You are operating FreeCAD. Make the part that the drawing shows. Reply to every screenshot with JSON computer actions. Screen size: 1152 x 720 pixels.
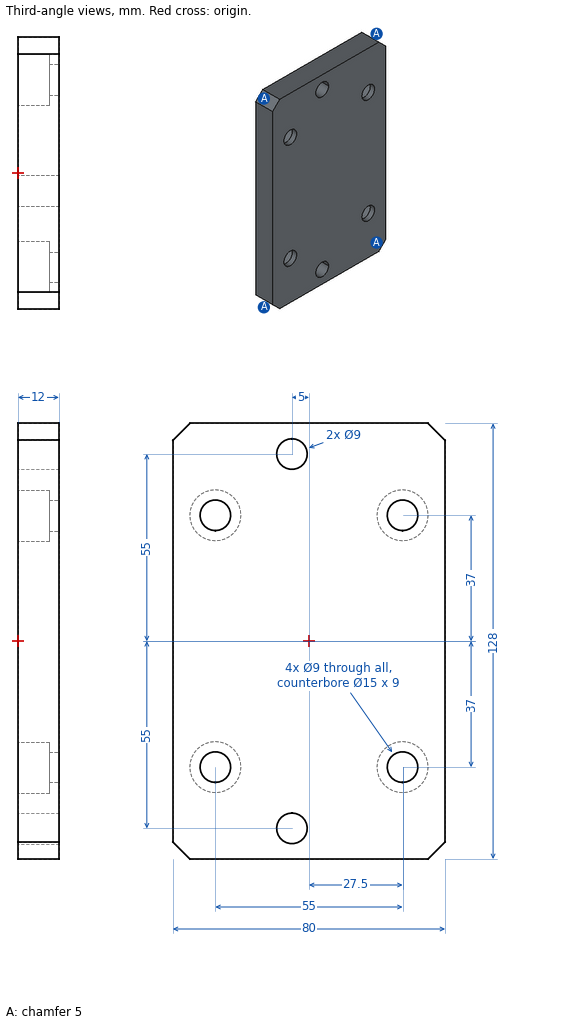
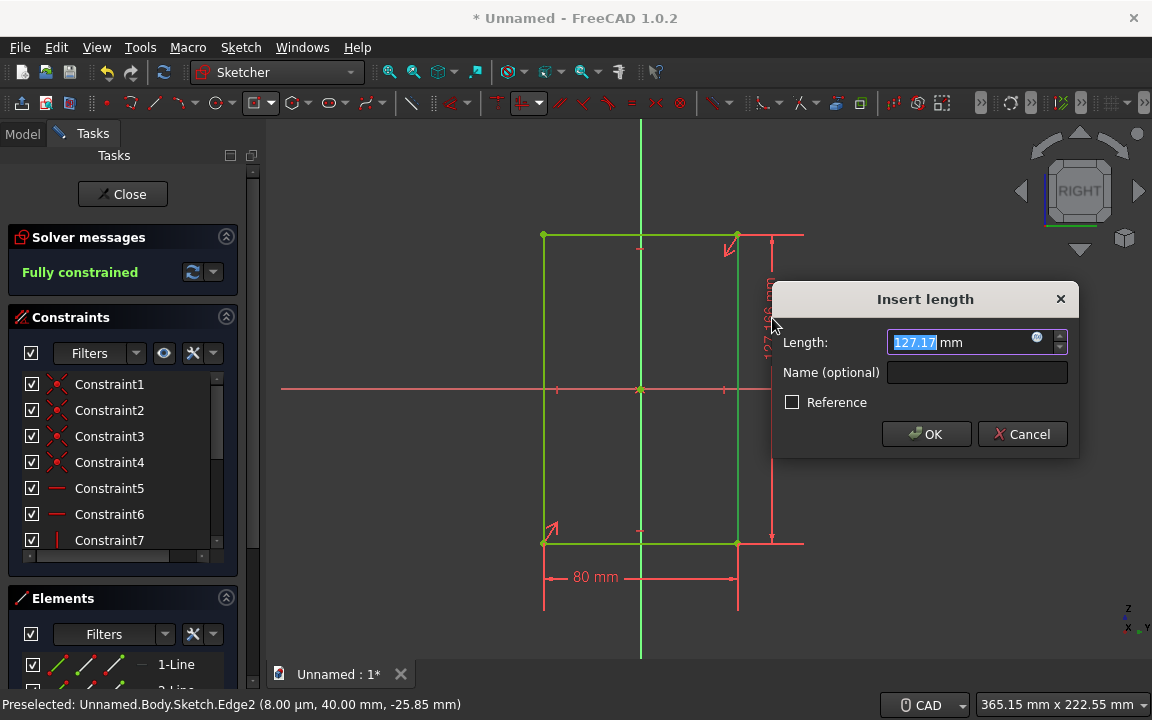
{"action": "type", "text": "128"}
{"action": "key", "text": "Return"}
{"action": "key", "text": "Escape"}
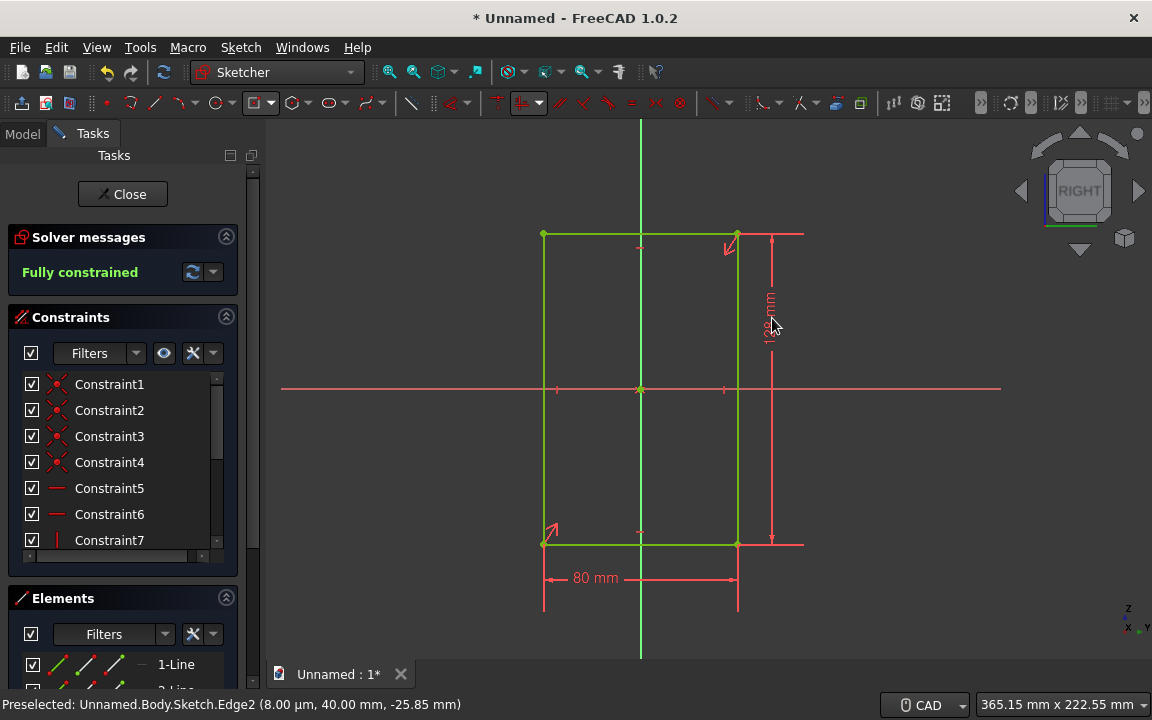
{"action": "left_click", "coordinate": [123, 194]}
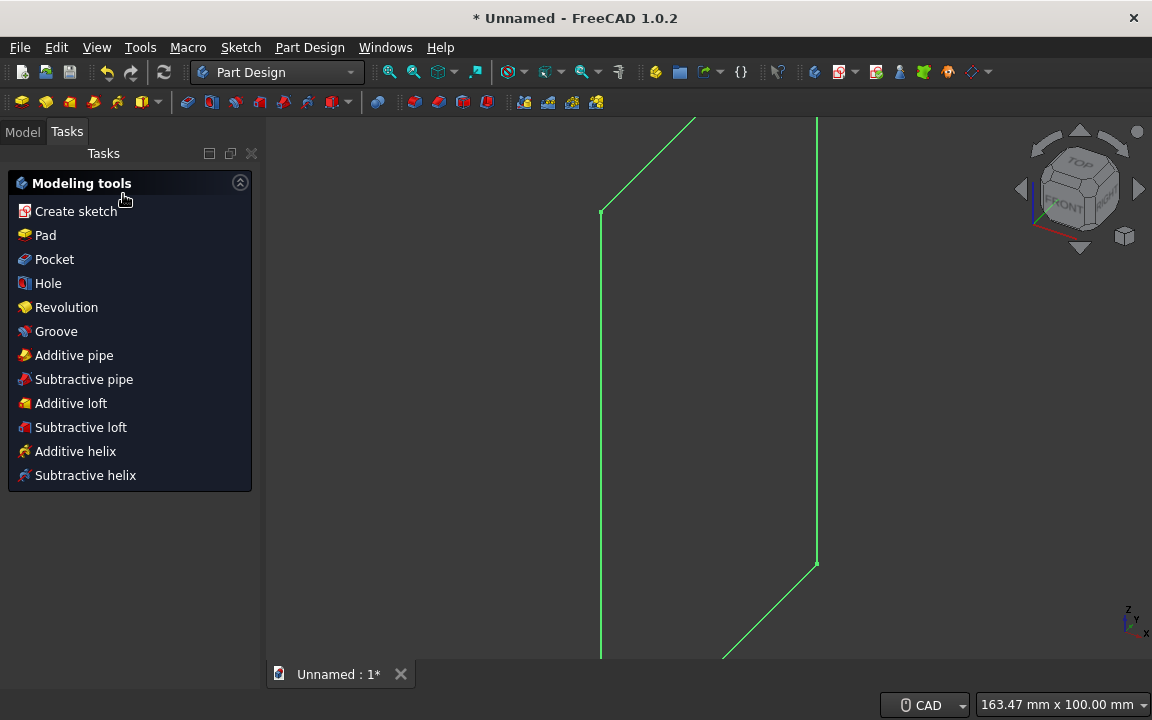
{"action": "left_click", "coordinate": [22, 102]}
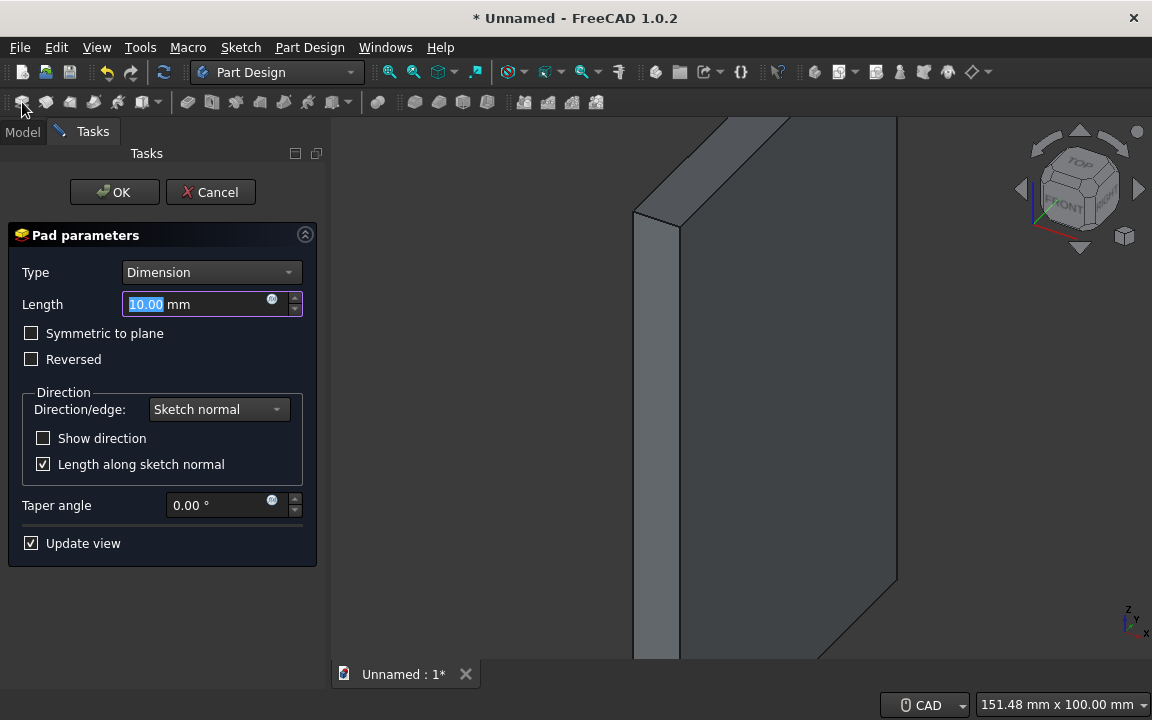
{"action": "type", "text": "12"}
{"action": "key", "text": "Tab"}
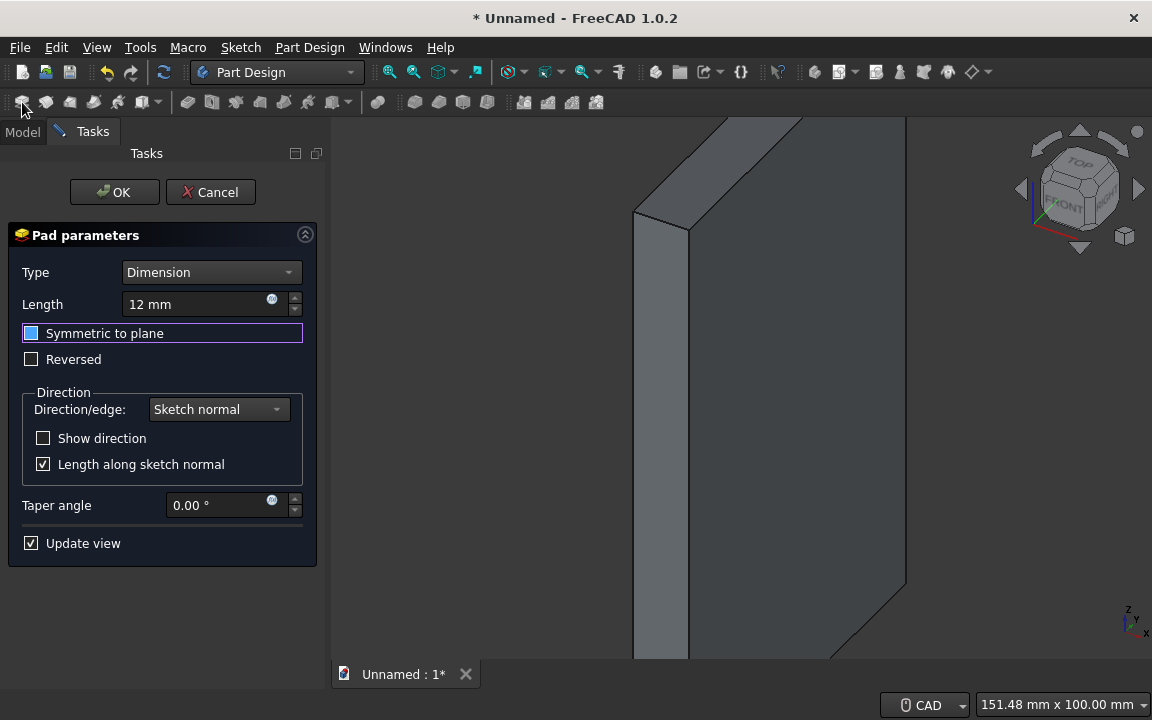
{"action": "left_click", "coordinate": [115, 192]}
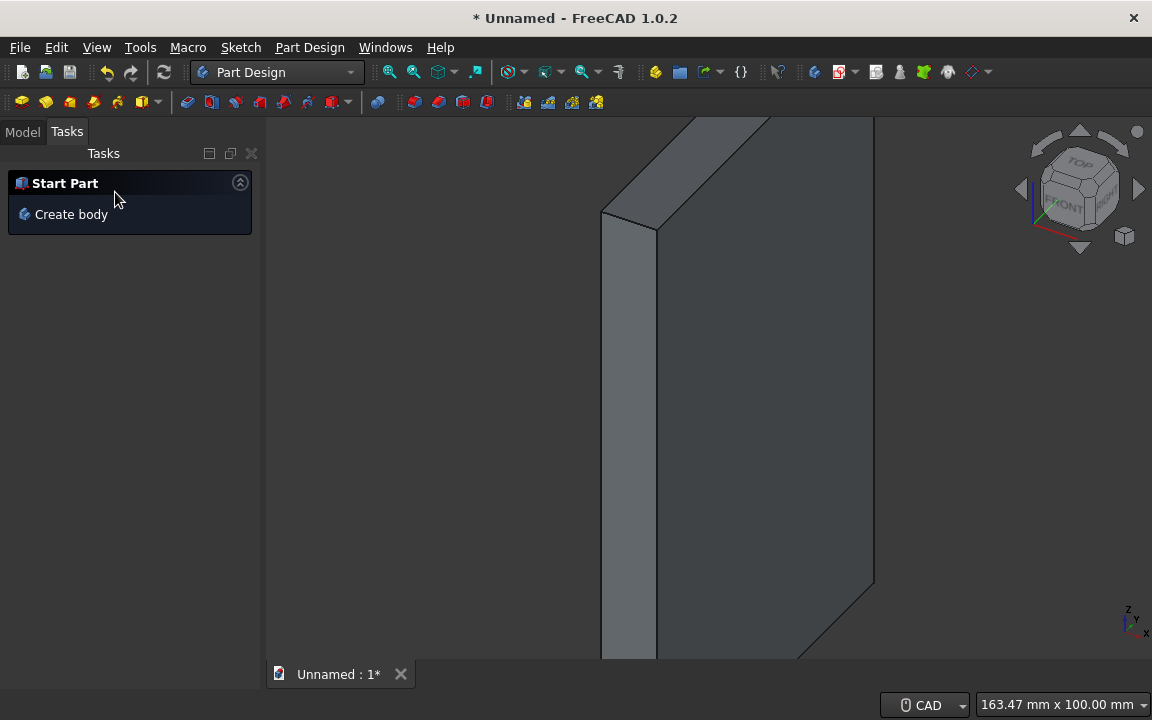
{"action": "left_click", "coordinate": [390, 72]}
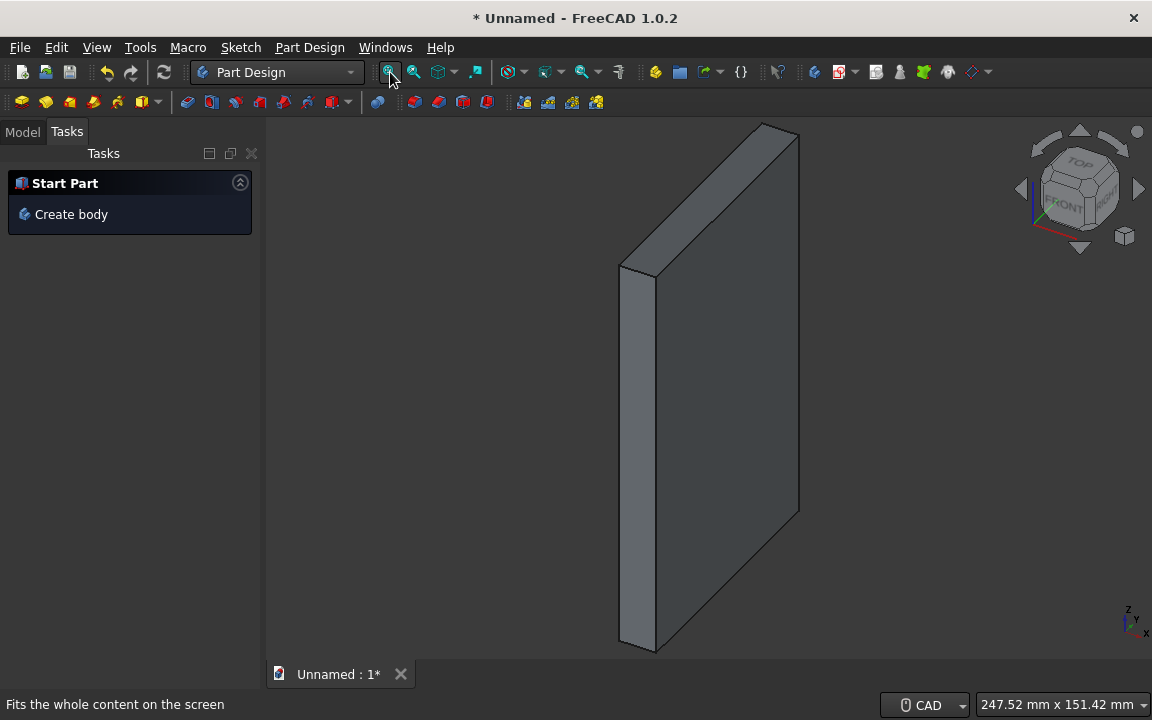
{"action": "left_click", "coordinate": [840, 72]}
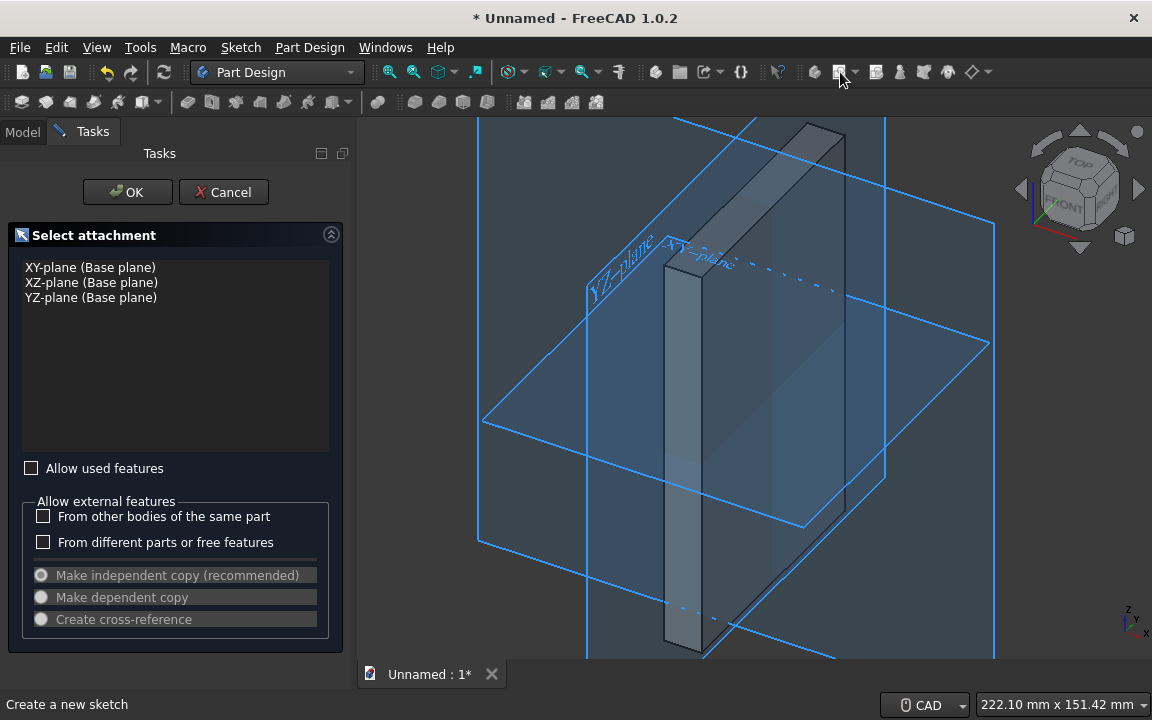
{"action": "left_click", "coordinate": [82, 298]}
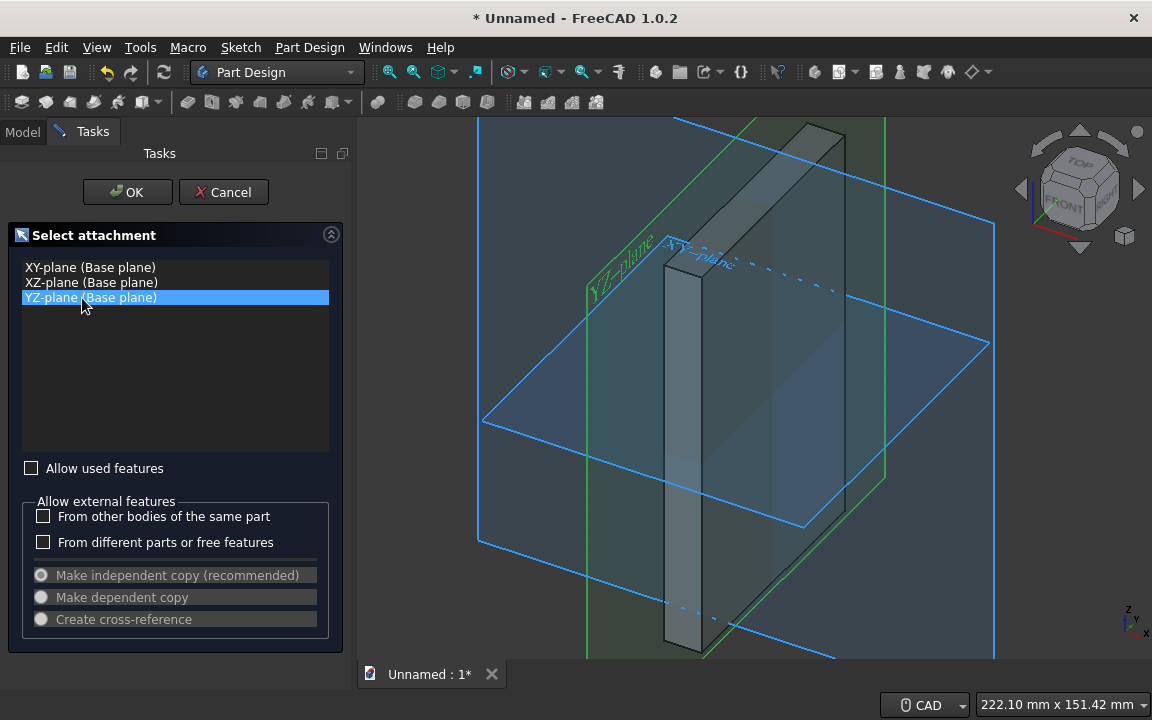
{"action": "left_click", "coordinate": [128, 192]}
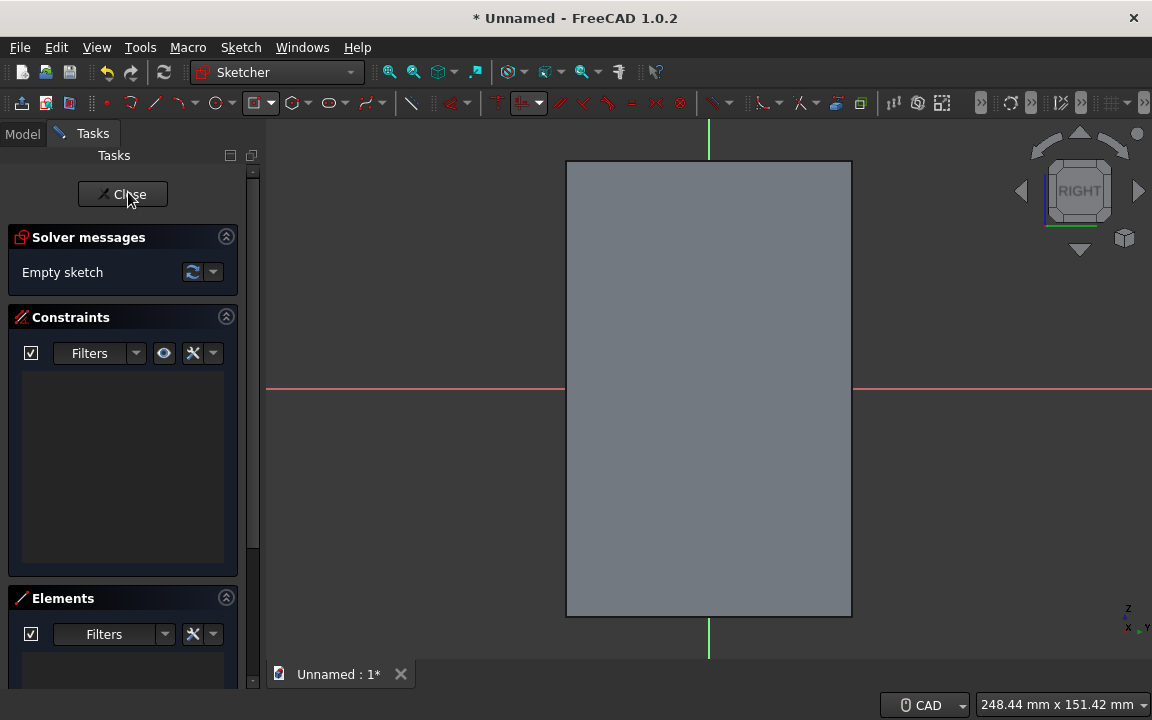
{"action": "left_click", "coordinate": [70, 104]}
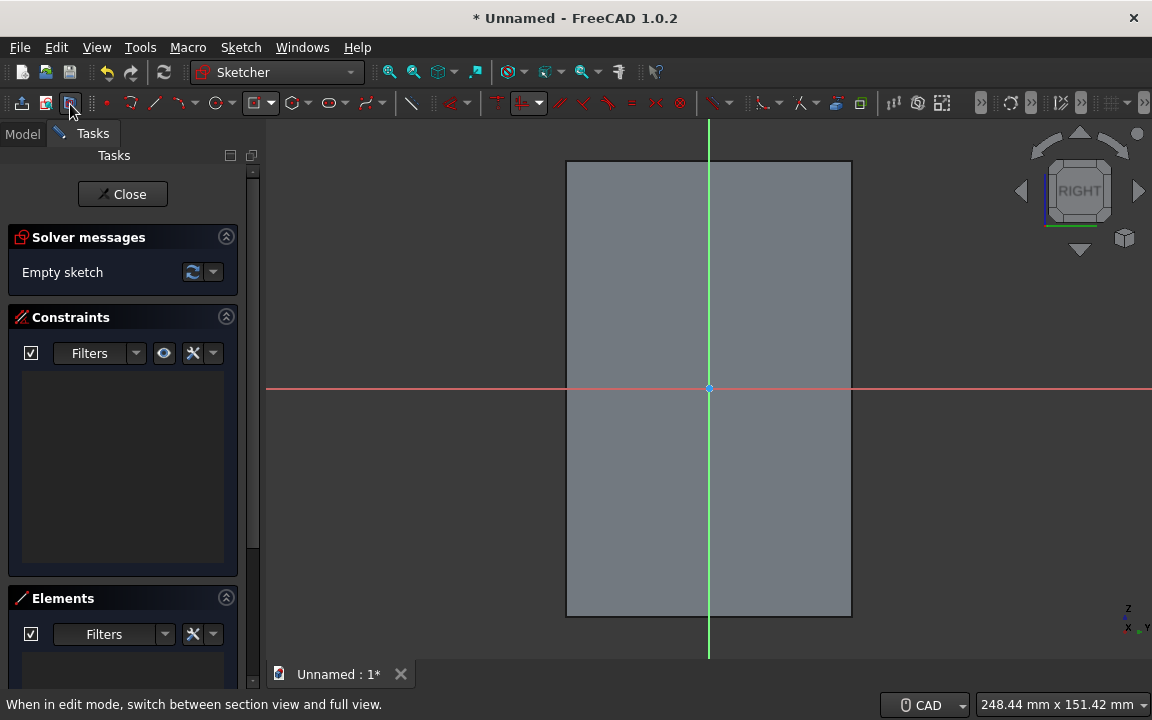
{"action": "left_click", "coordinate": [216, 104]}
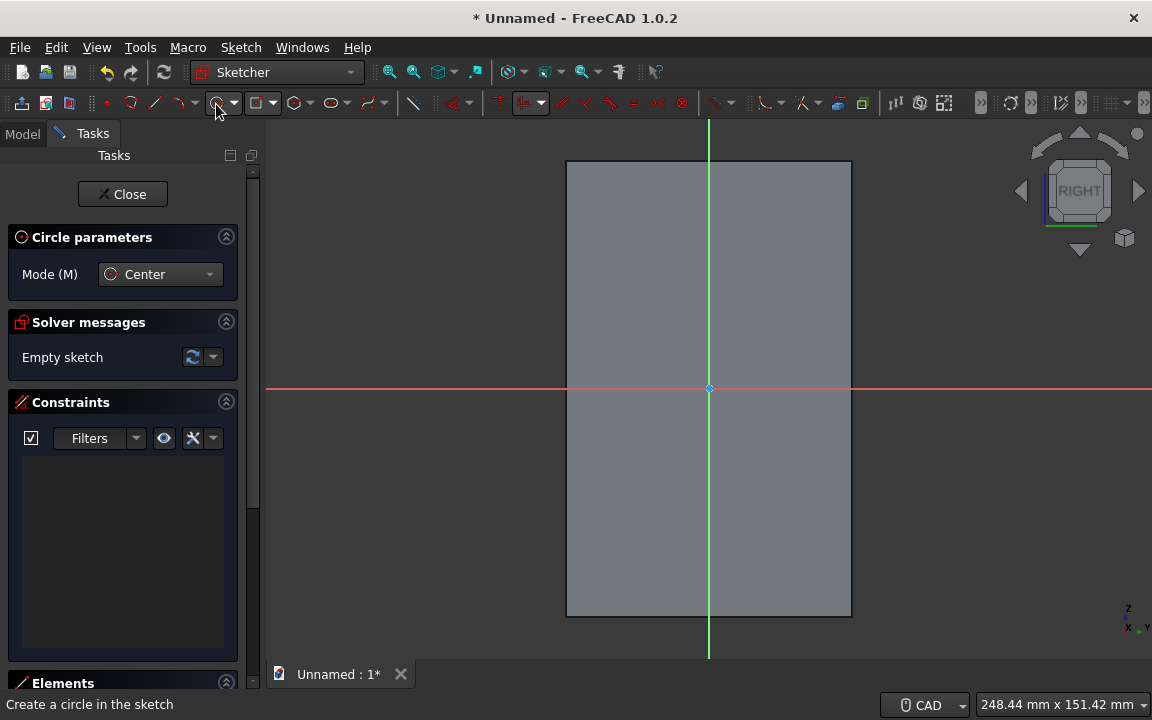
{"action": "scroll", "coordinate": [807, 521], "scroll_direction": "up", "scroll_amount": 2}